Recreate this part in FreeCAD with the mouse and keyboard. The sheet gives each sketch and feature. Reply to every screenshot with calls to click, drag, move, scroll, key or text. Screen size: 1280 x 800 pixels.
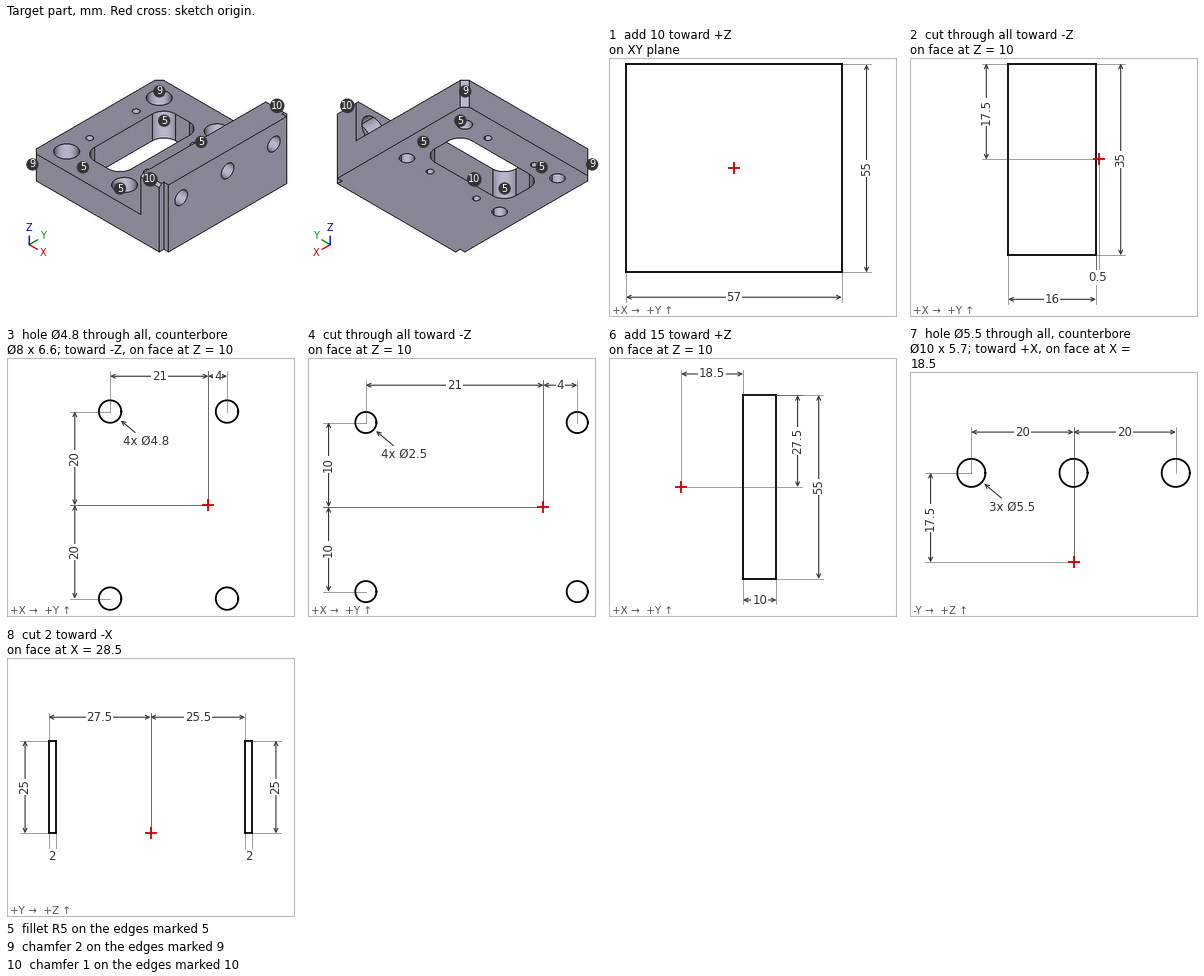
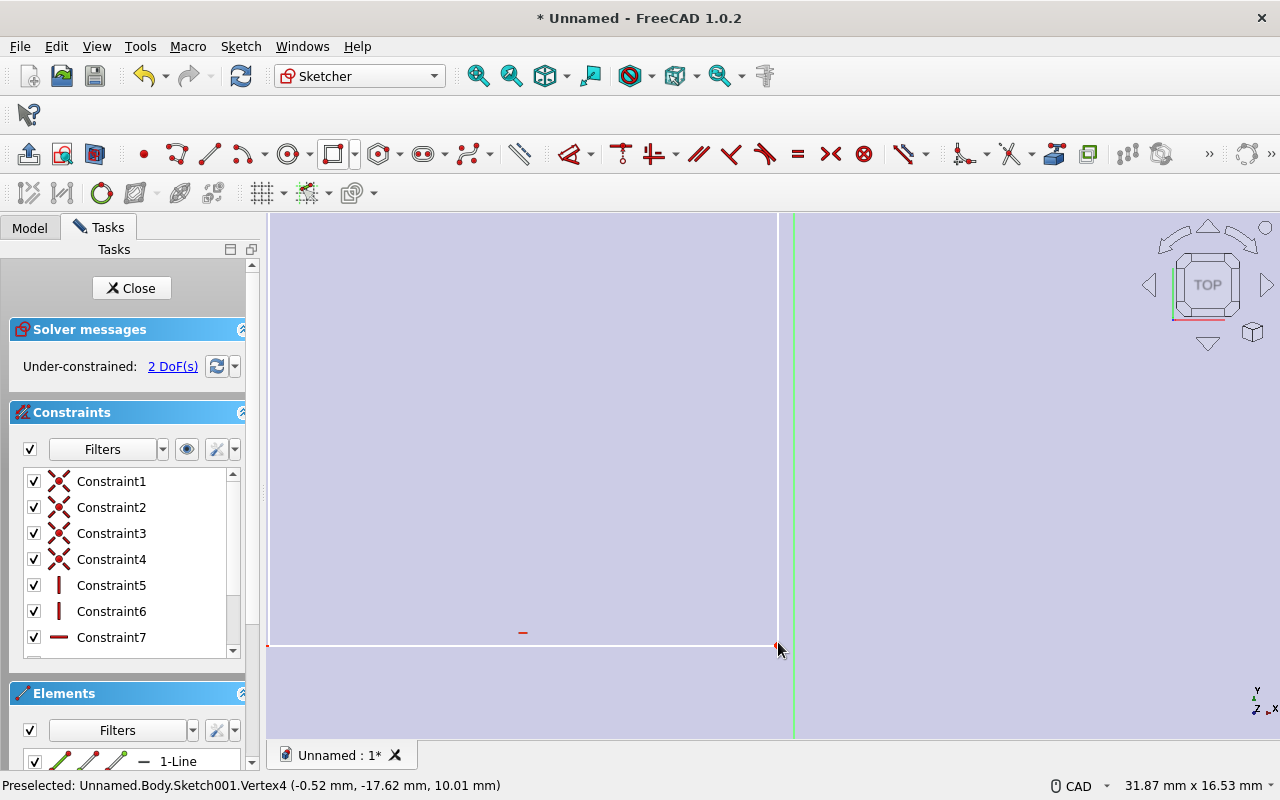
scroll(778, 646, up, 5)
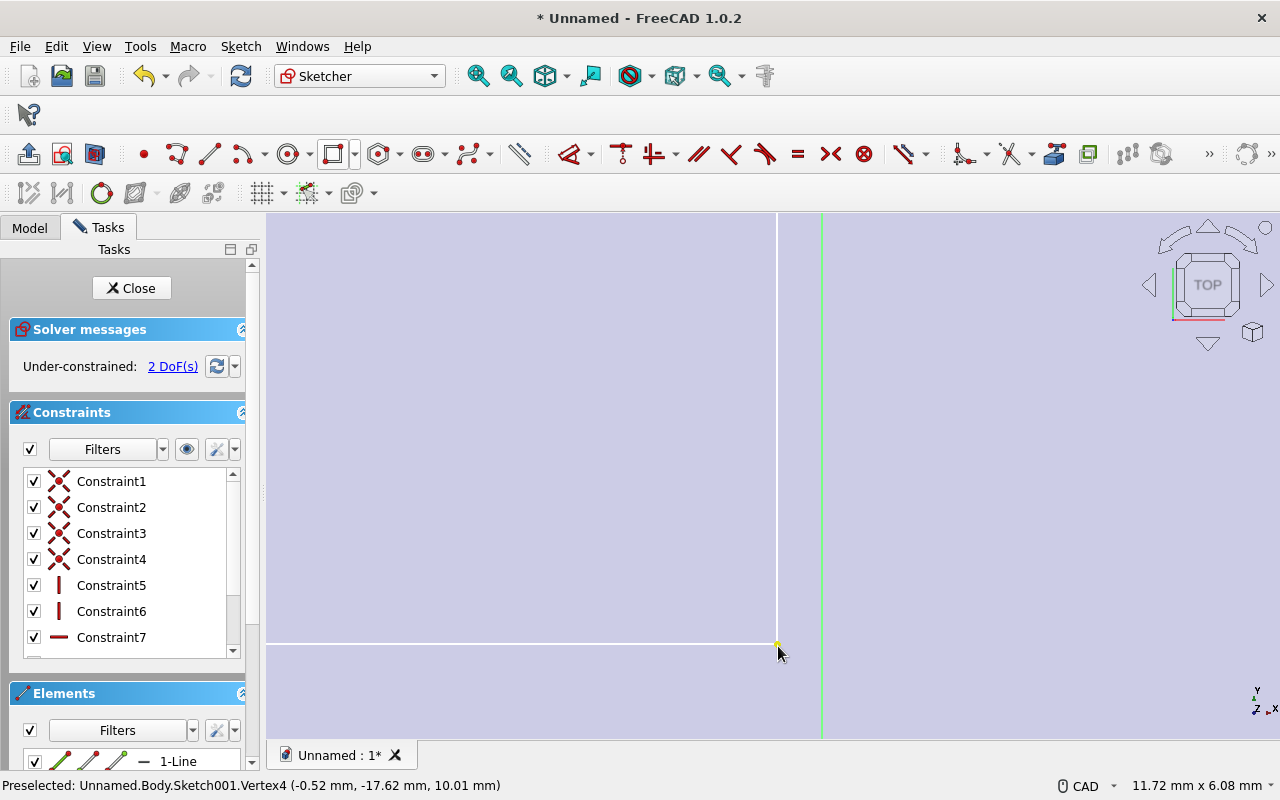
click(777, 644)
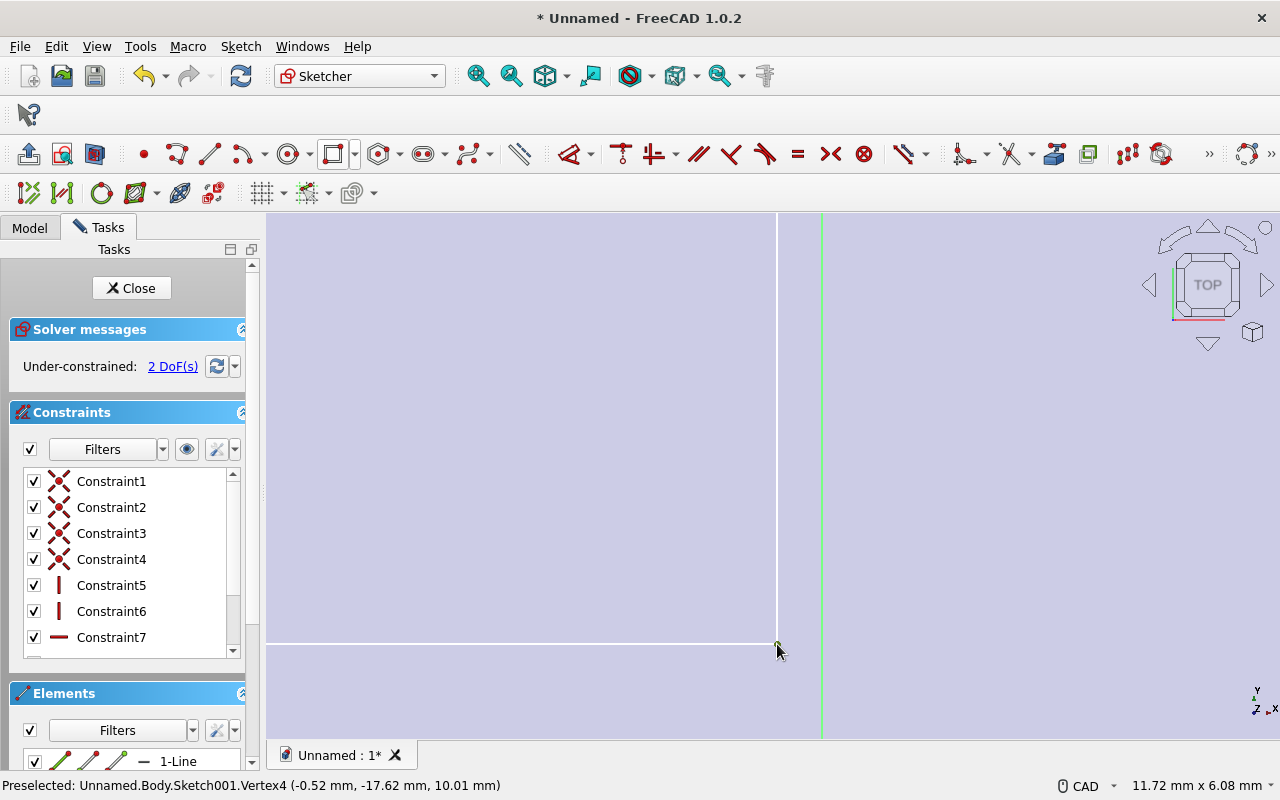
key(l)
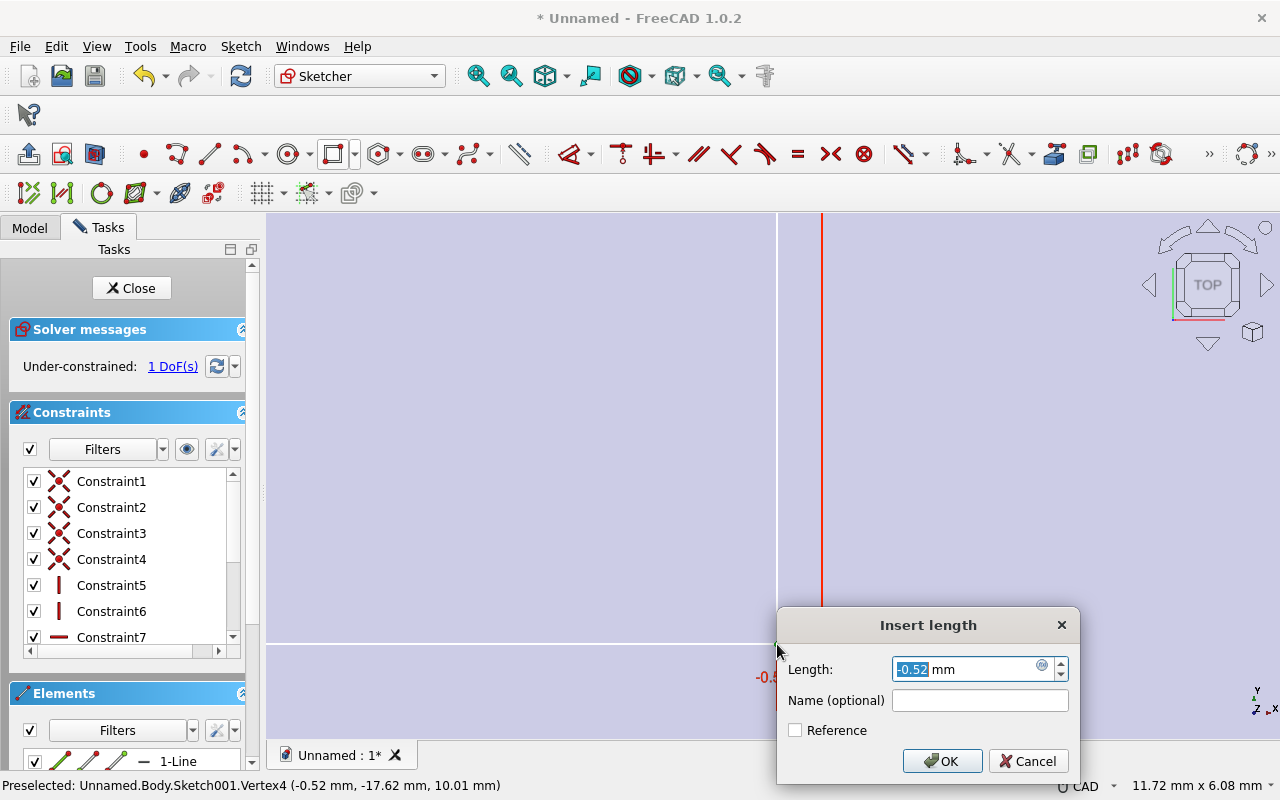
text(-0.5)
key(Return)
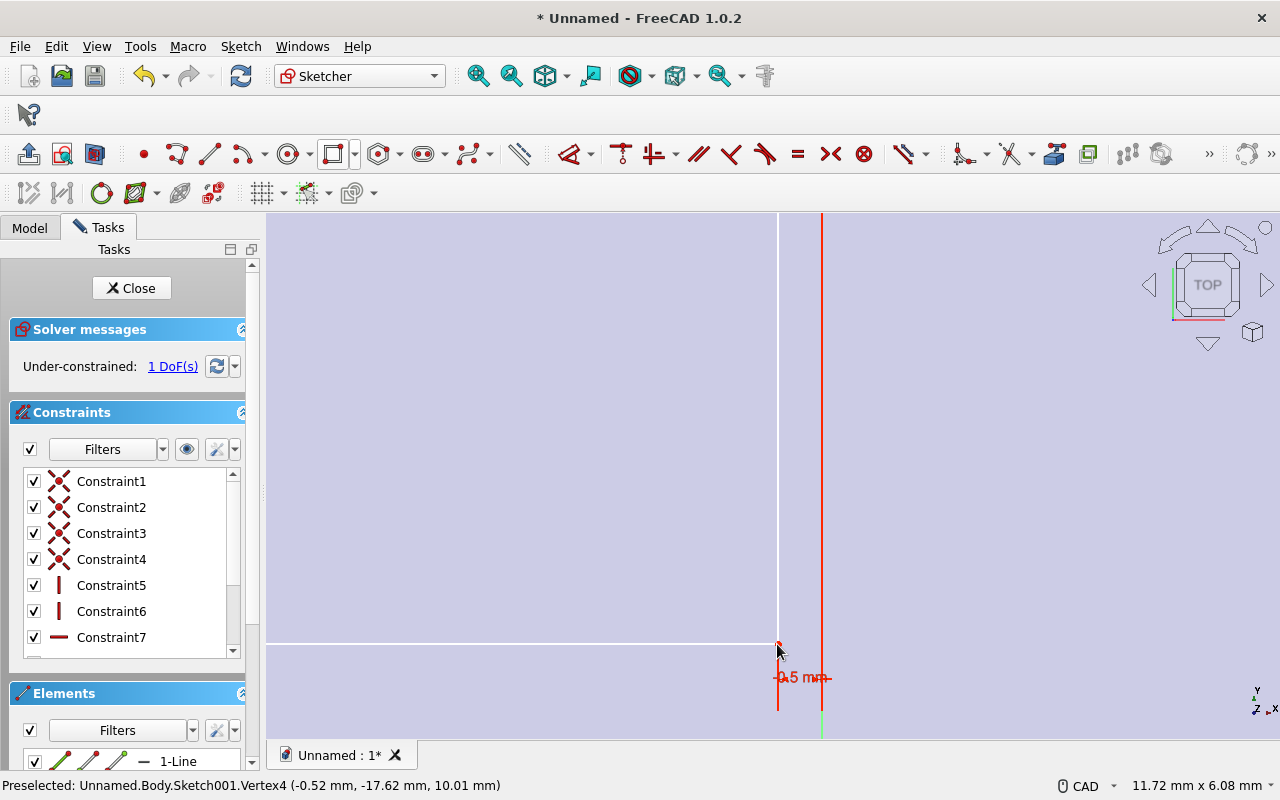
scroll(779, 645, down, 11)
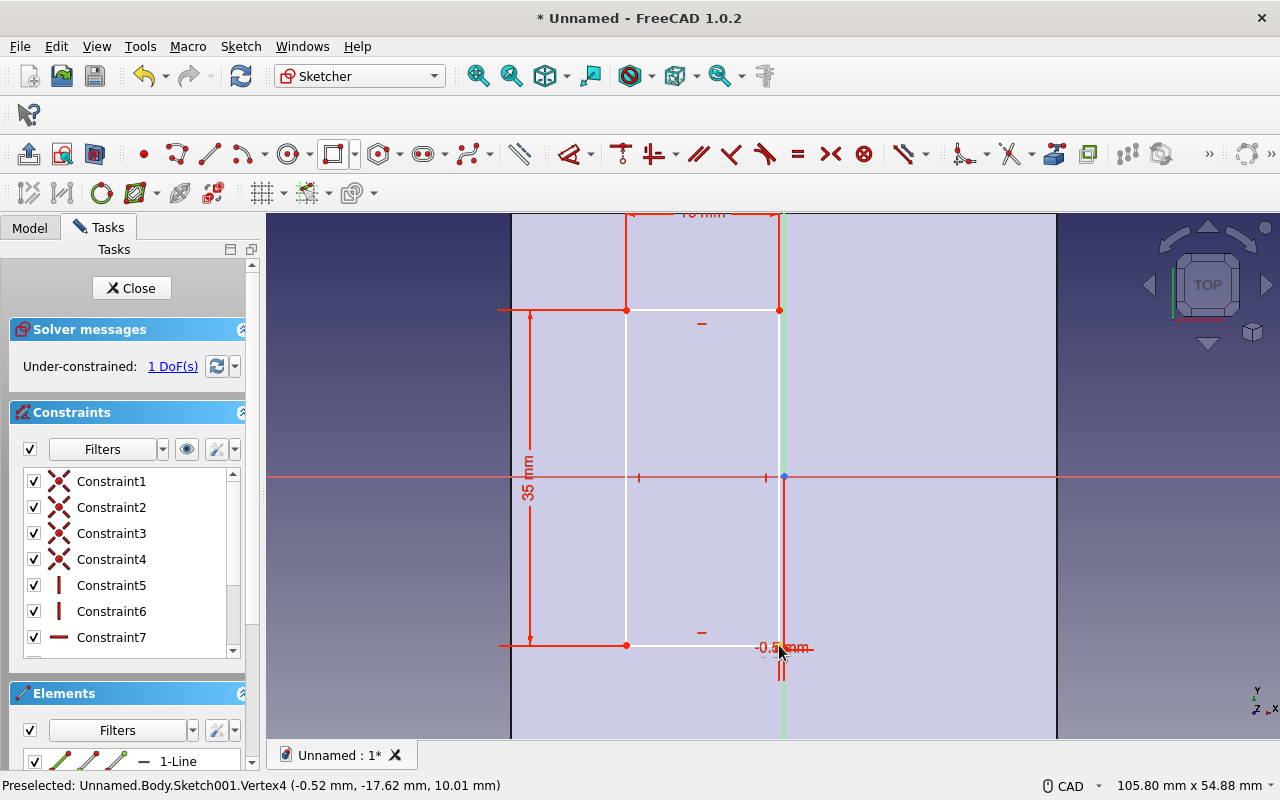
click(626, 310)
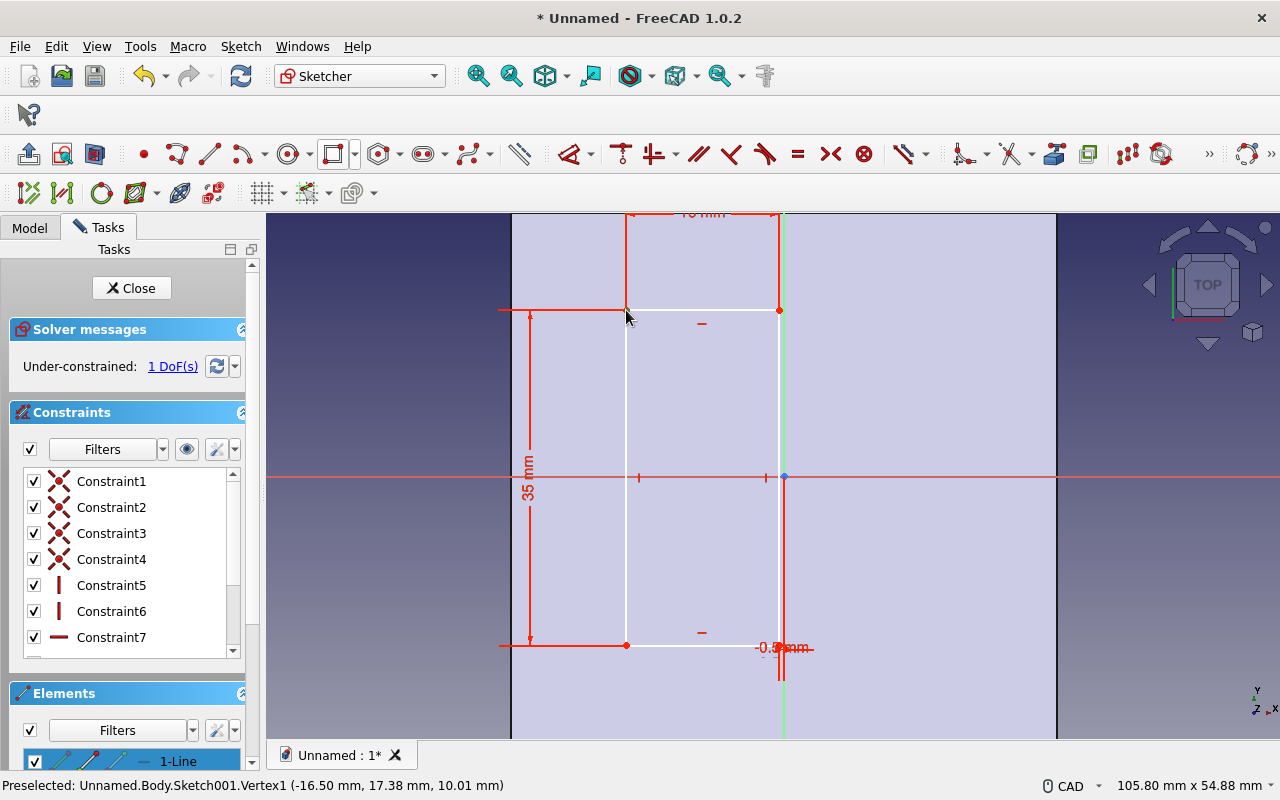
key(i)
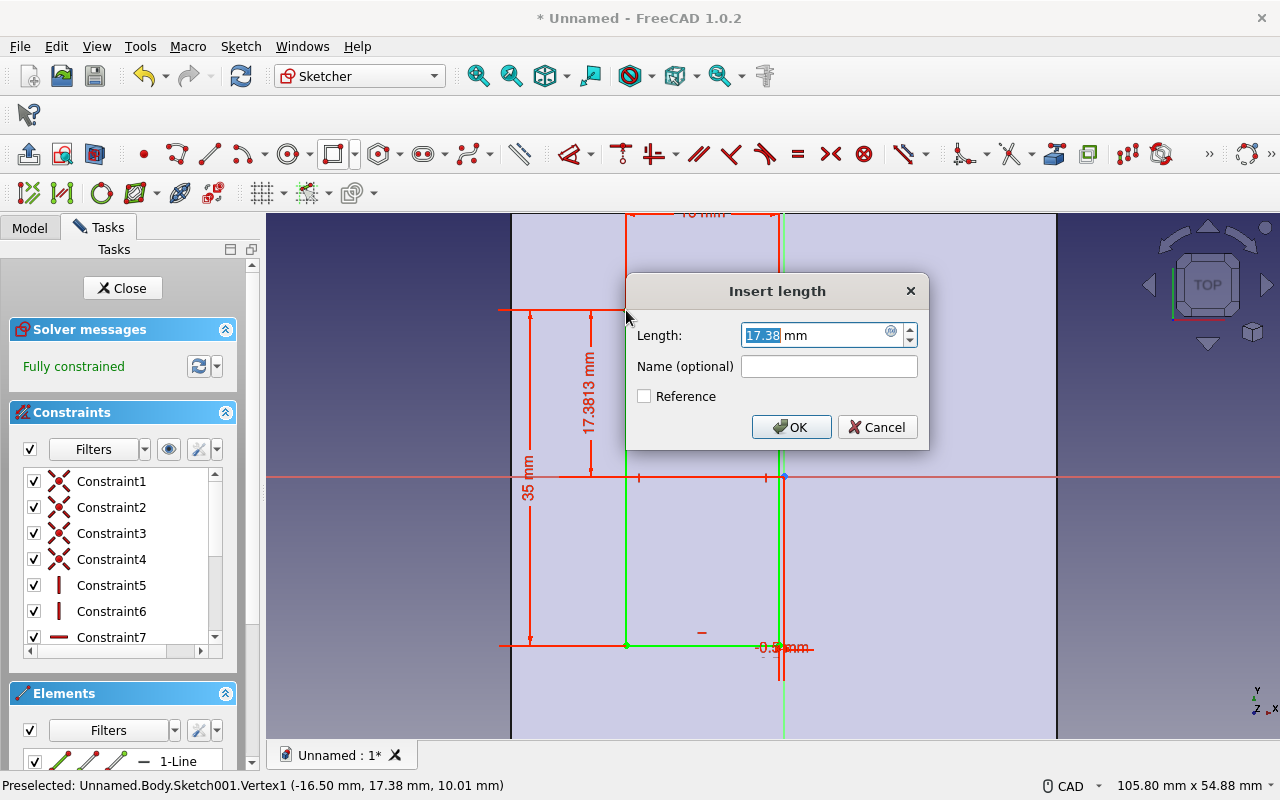
text(17.5)
key(Return)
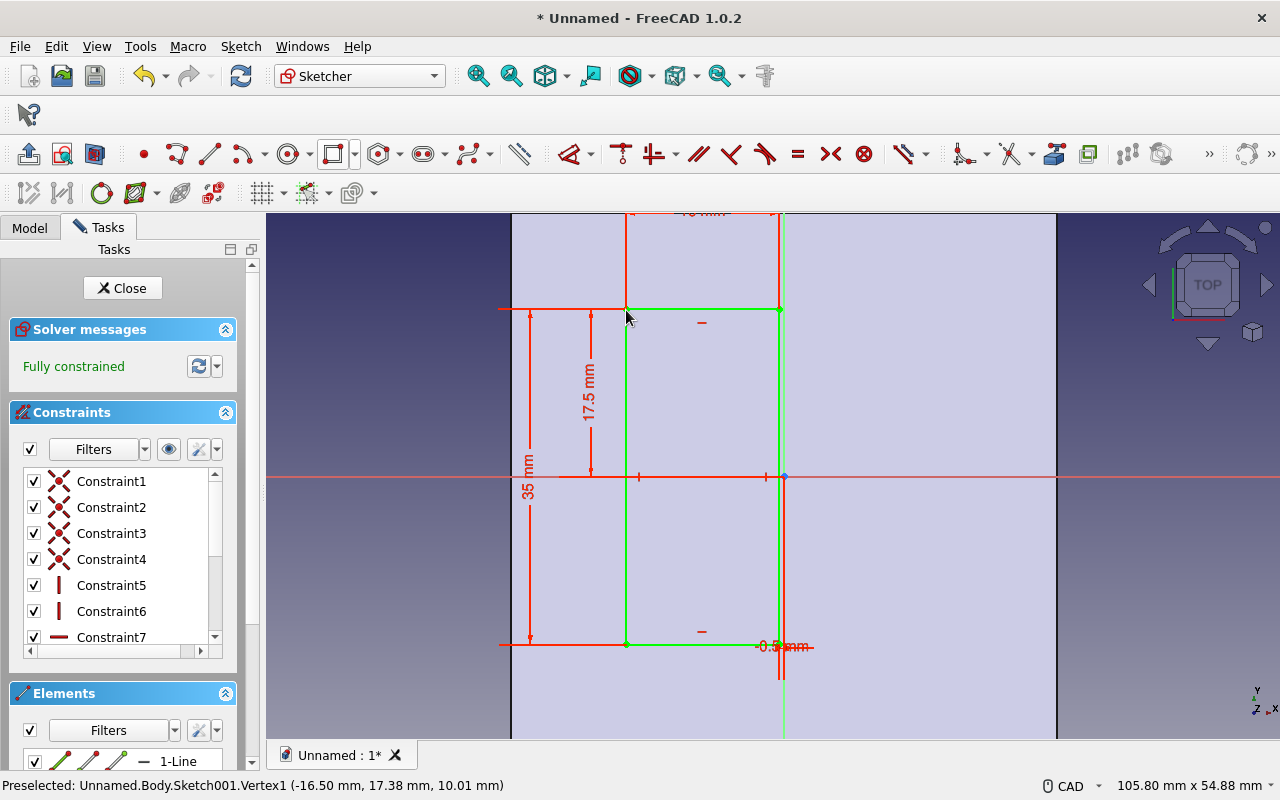
click(123, 288)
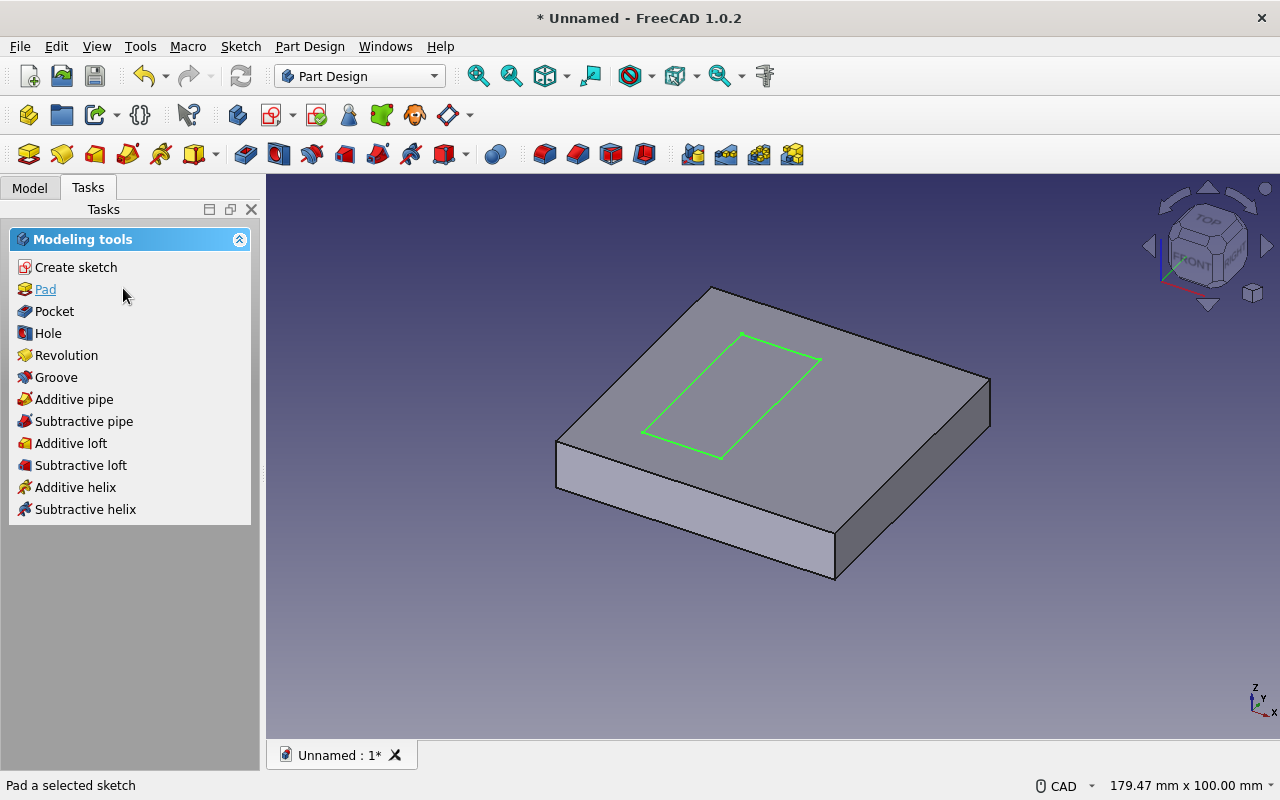
click(246, 154)